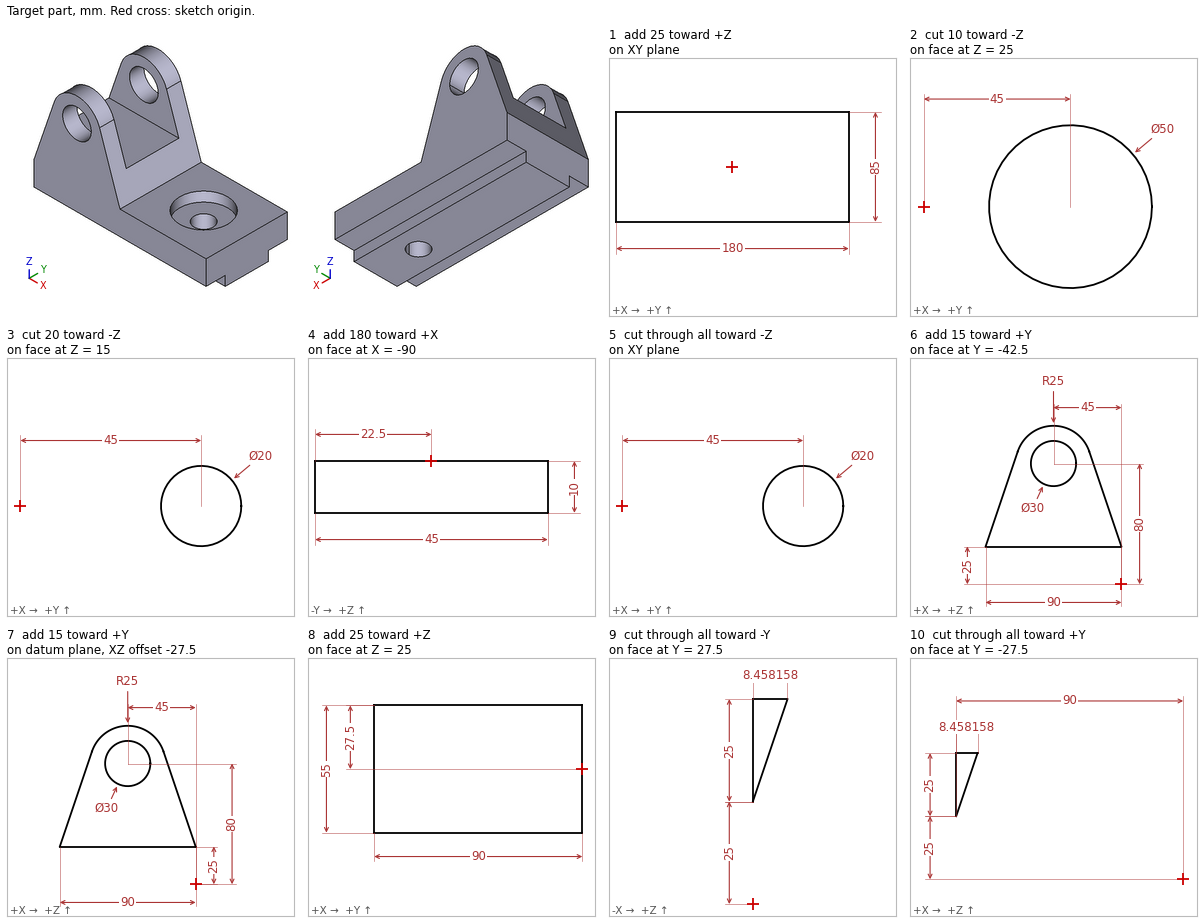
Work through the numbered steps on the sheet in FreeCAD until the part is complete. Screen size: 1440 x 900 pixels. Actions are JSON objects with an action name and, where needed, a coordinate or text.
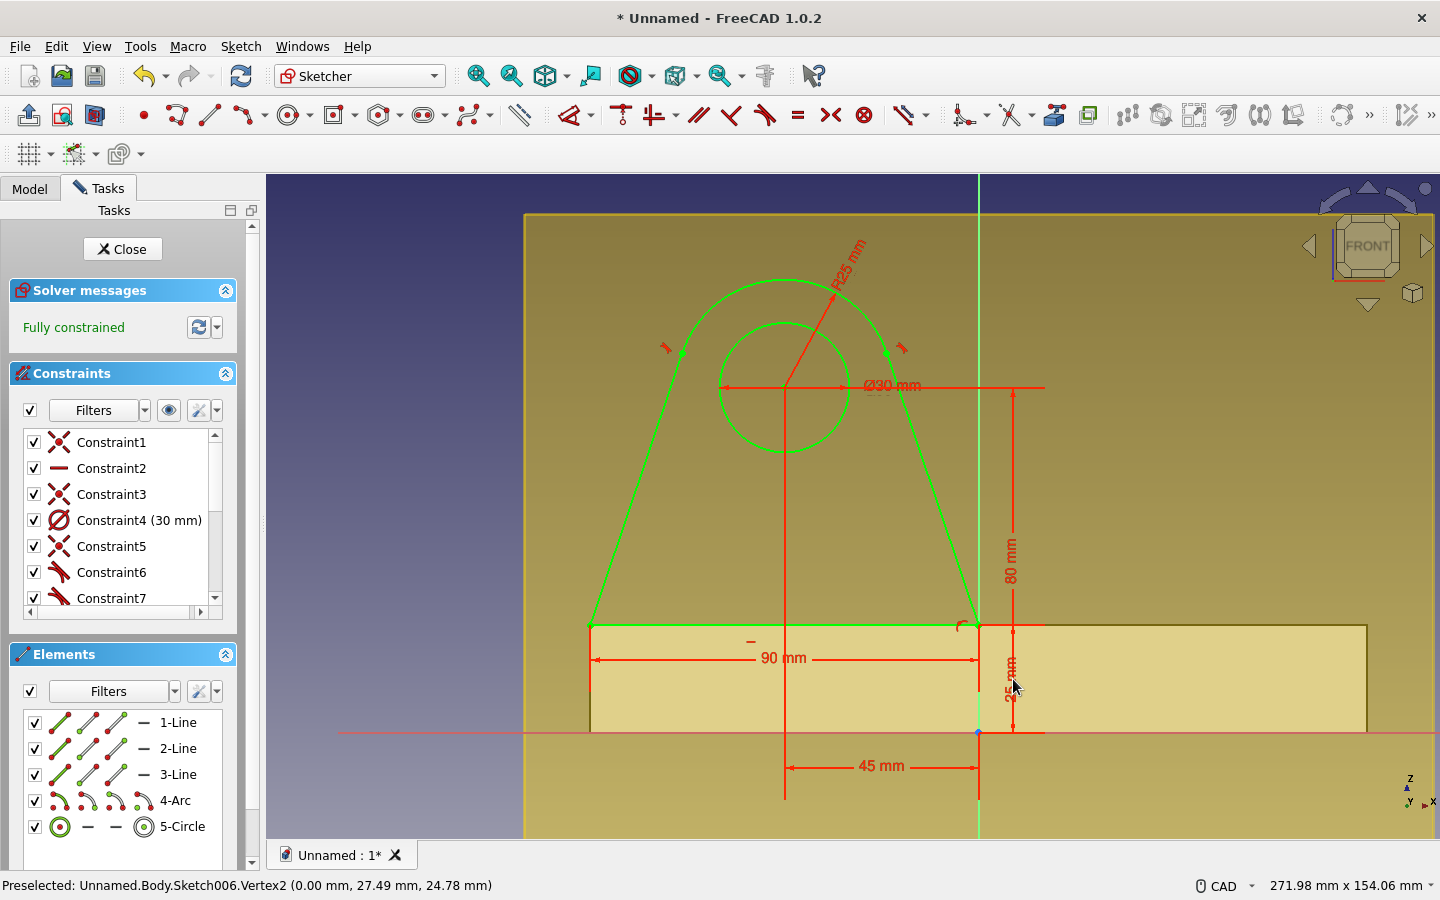
{"action": "left_click", "coordinate": [123, 249]}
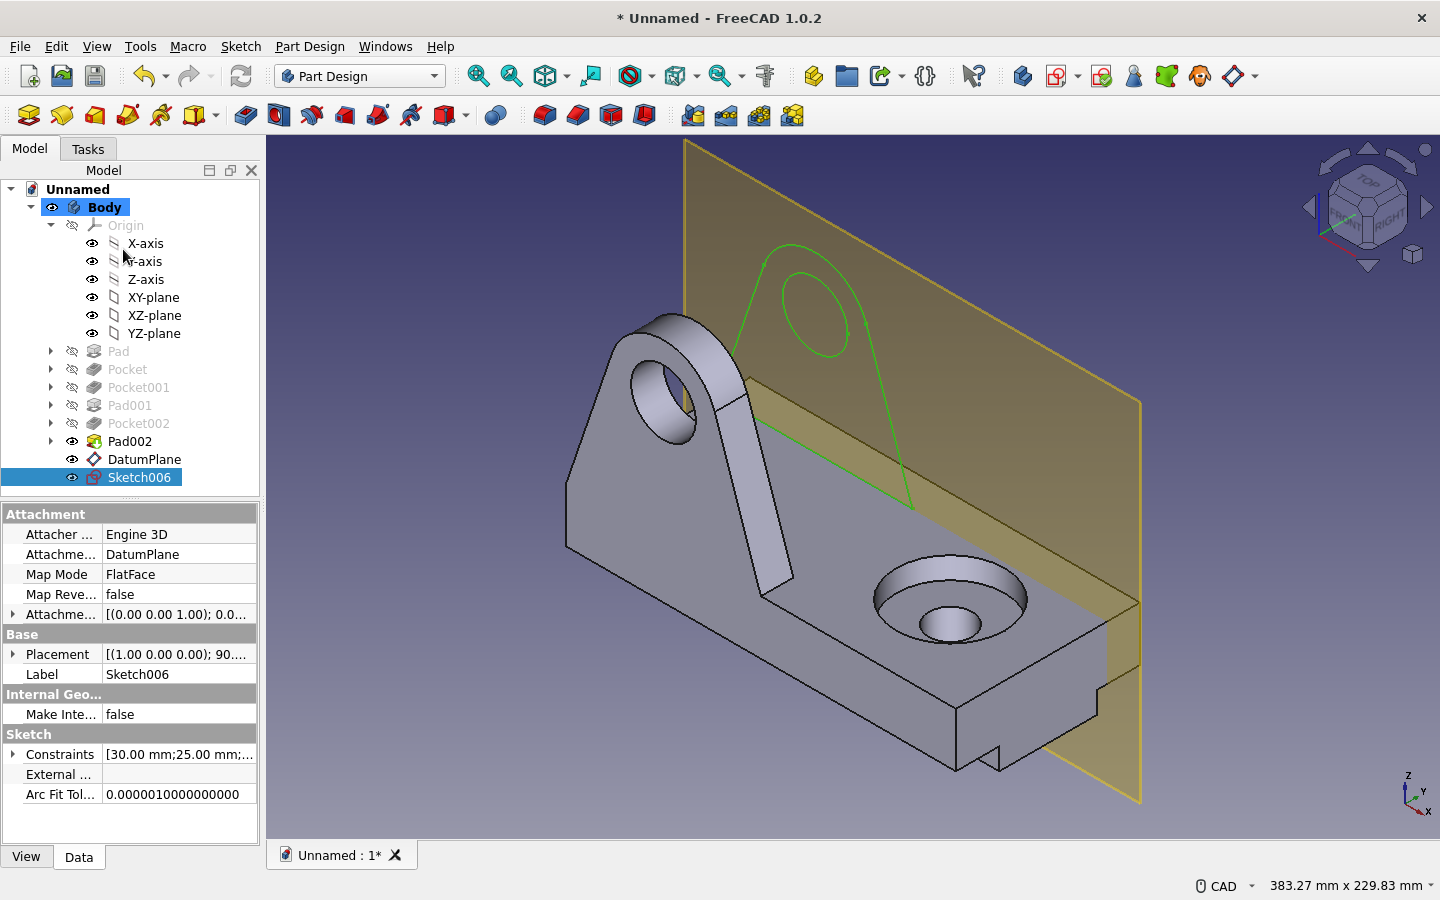
{"action": "left_click", "coordinate": [29, 116]}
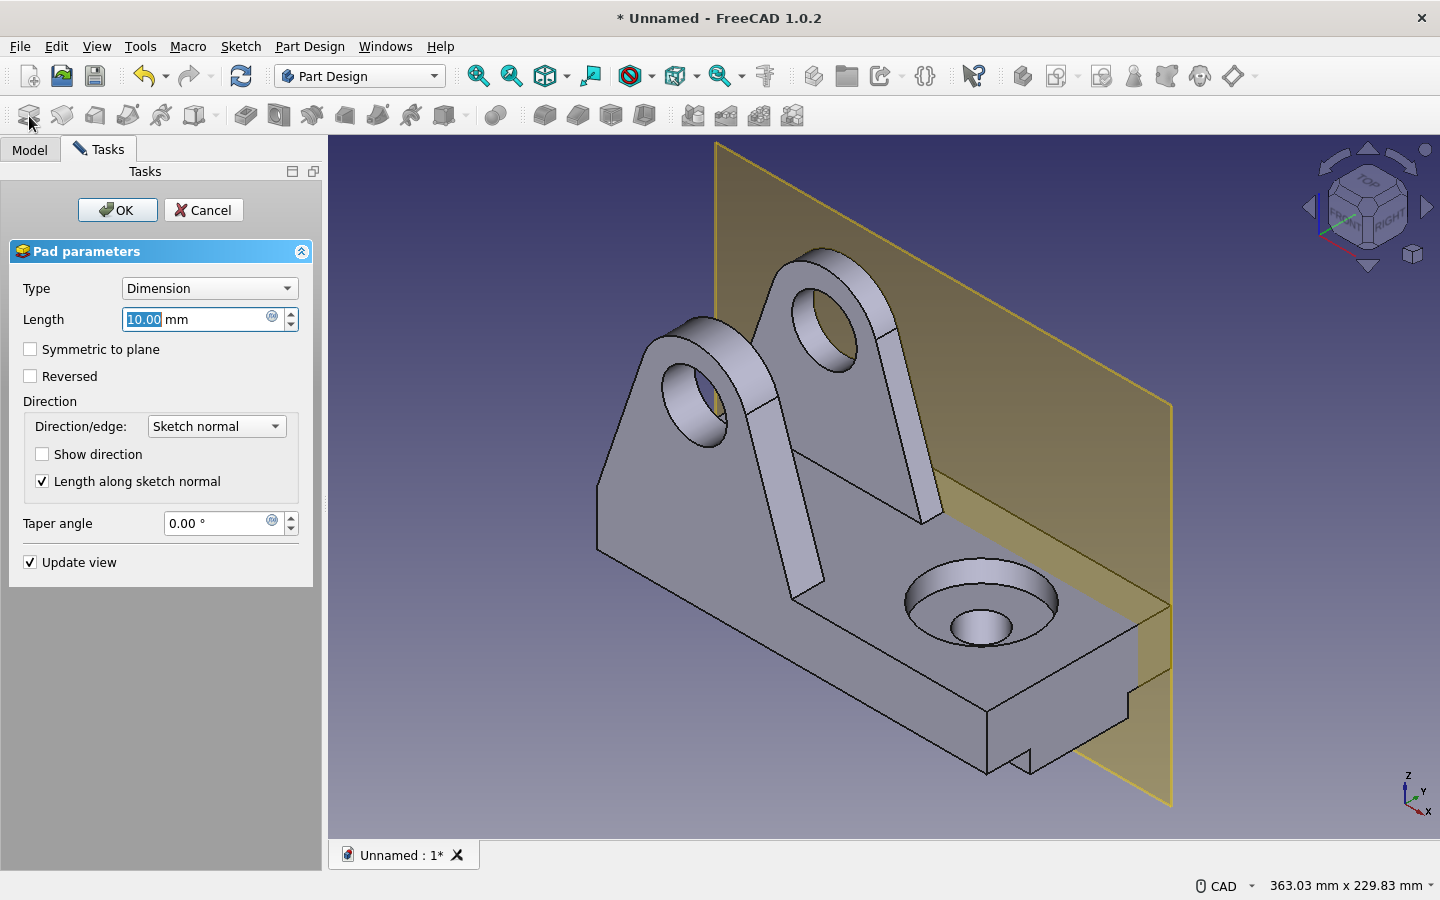
{"action": "type", "text": "15"}
{"action": "key", "text": "Tab"}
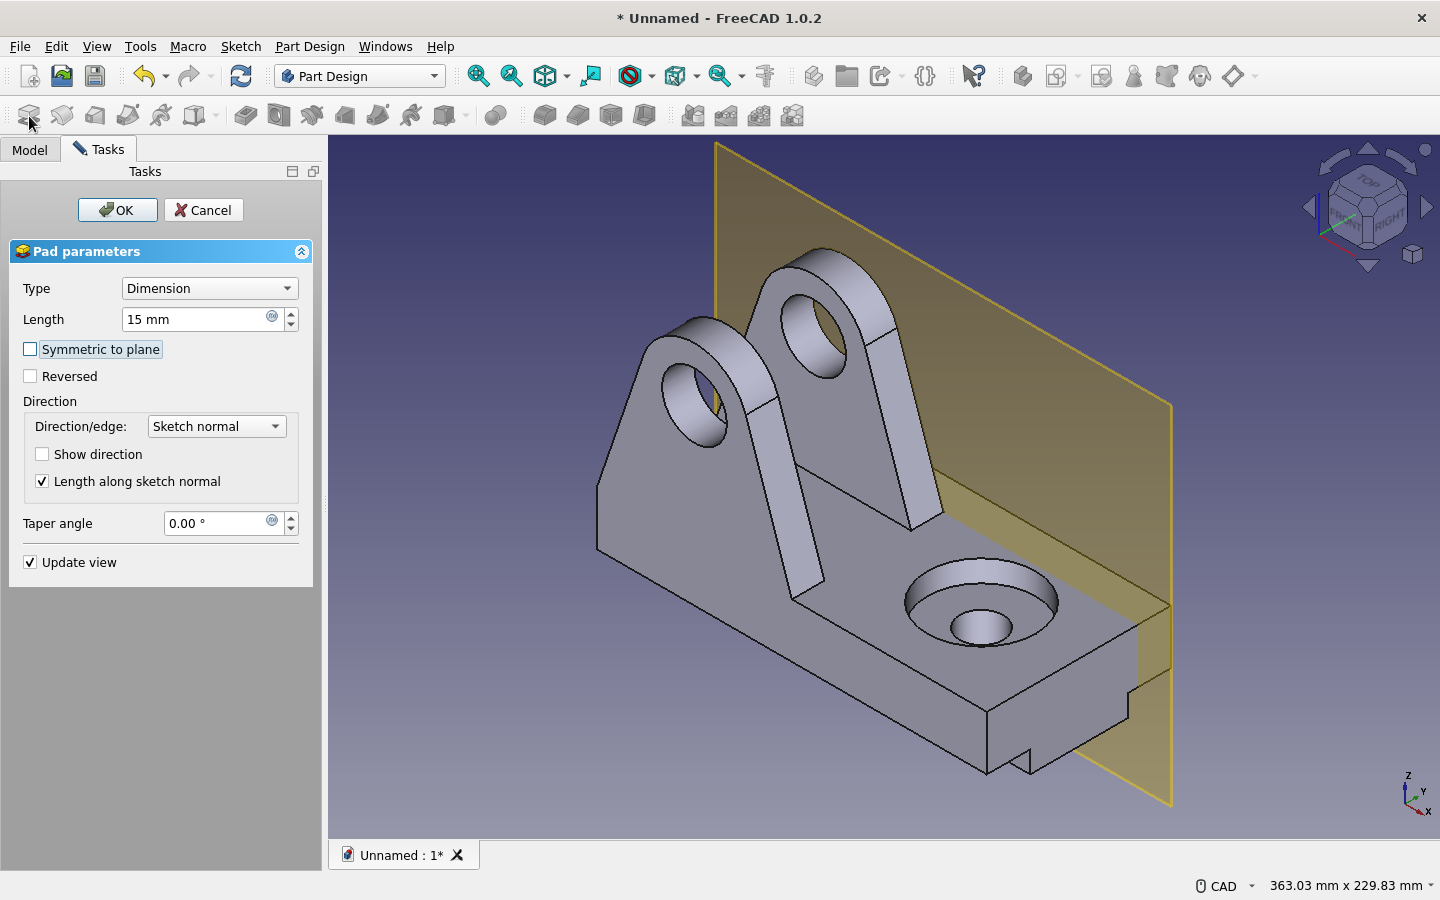
{"action": "left_click", "coordinate": [31, 376]}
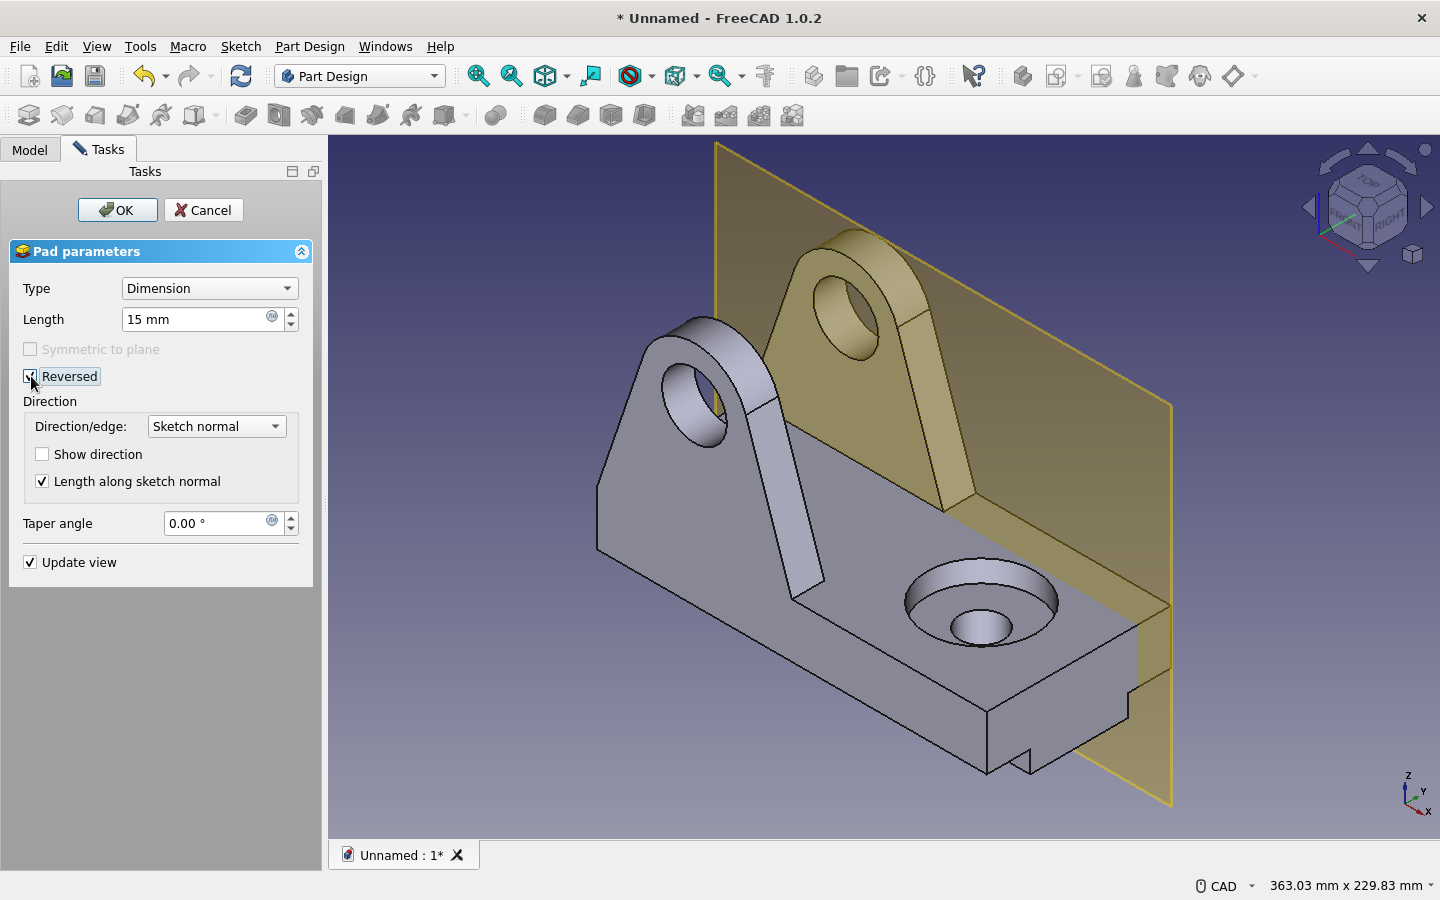
{"action": "left_click", "coordinate": [118, 210]}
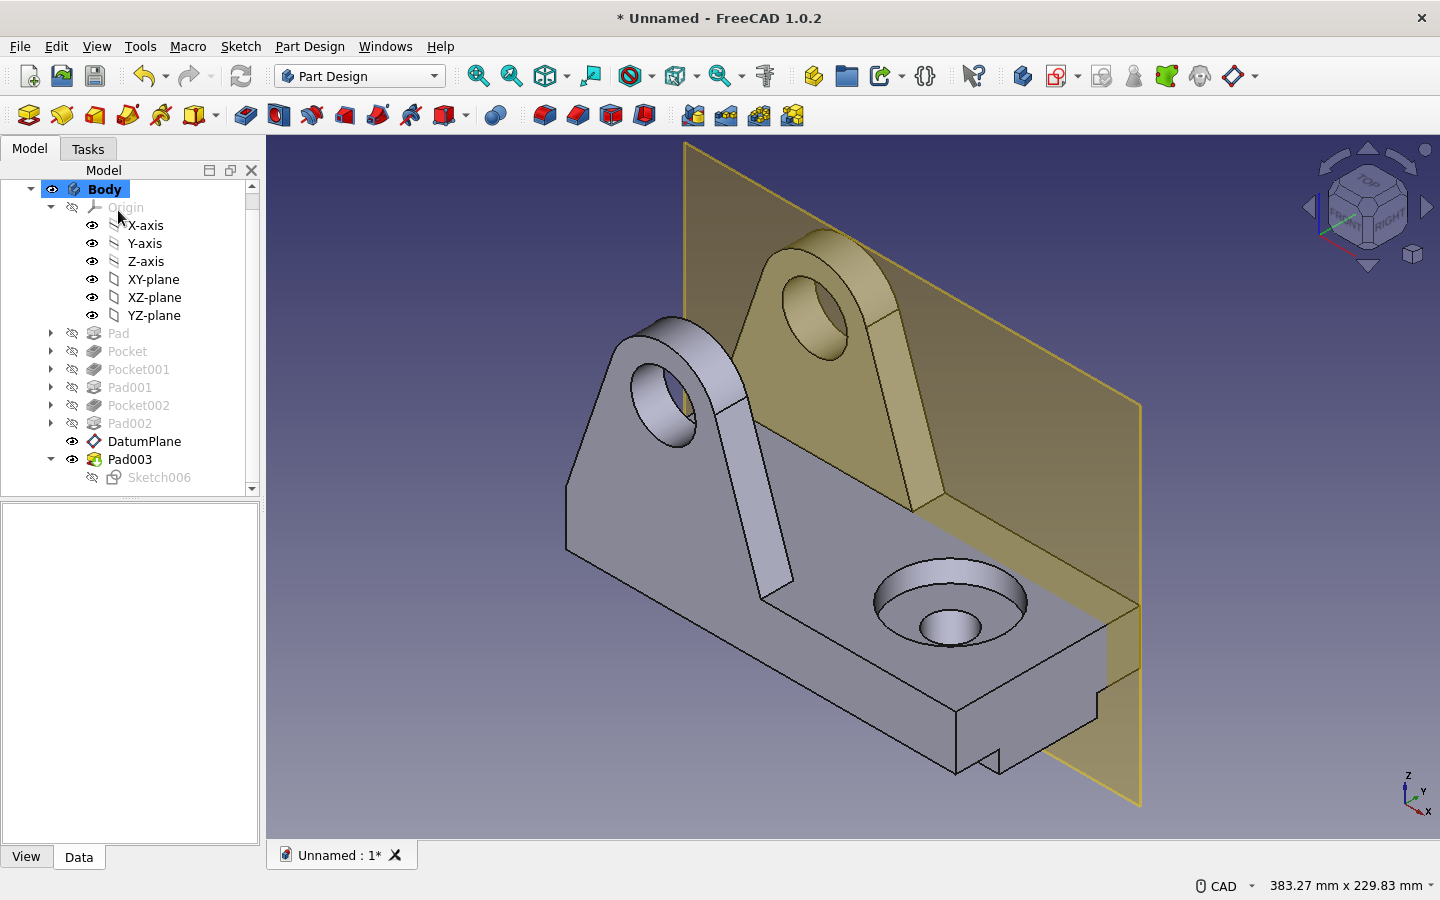
{"action": "left_click", "coordinate": [117, 441]}
{"action": "key", "text": "space"}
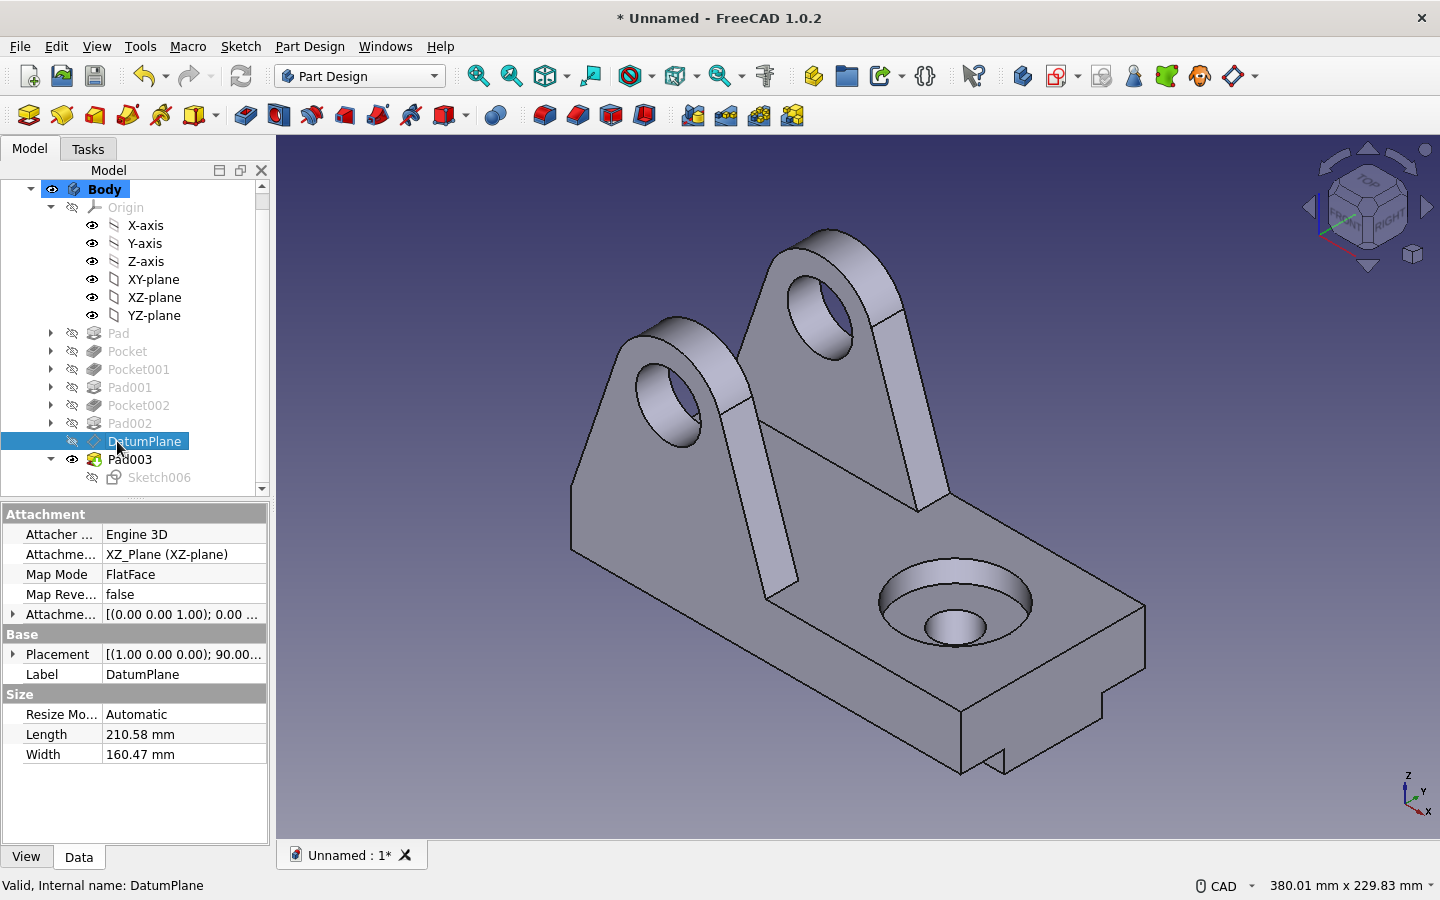
{"action": "left_click", "coordinate": [802, 513]}